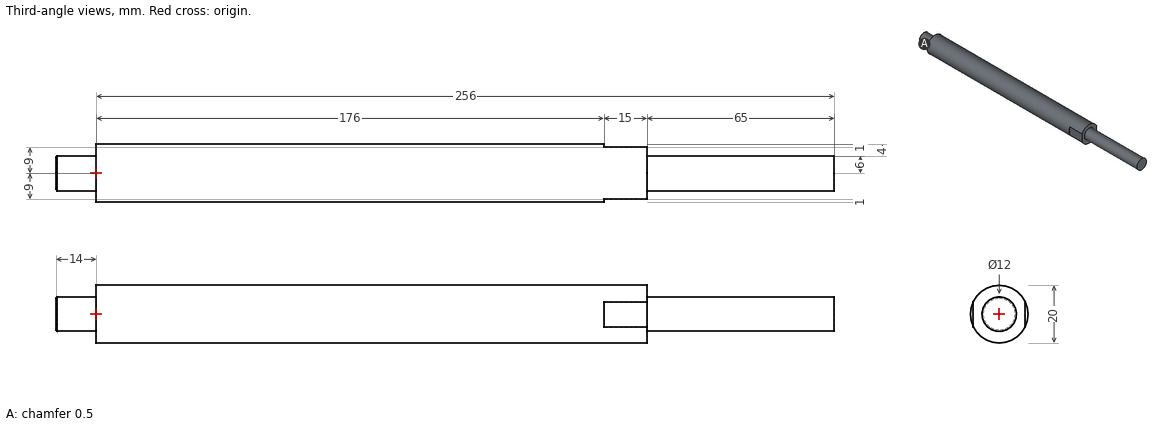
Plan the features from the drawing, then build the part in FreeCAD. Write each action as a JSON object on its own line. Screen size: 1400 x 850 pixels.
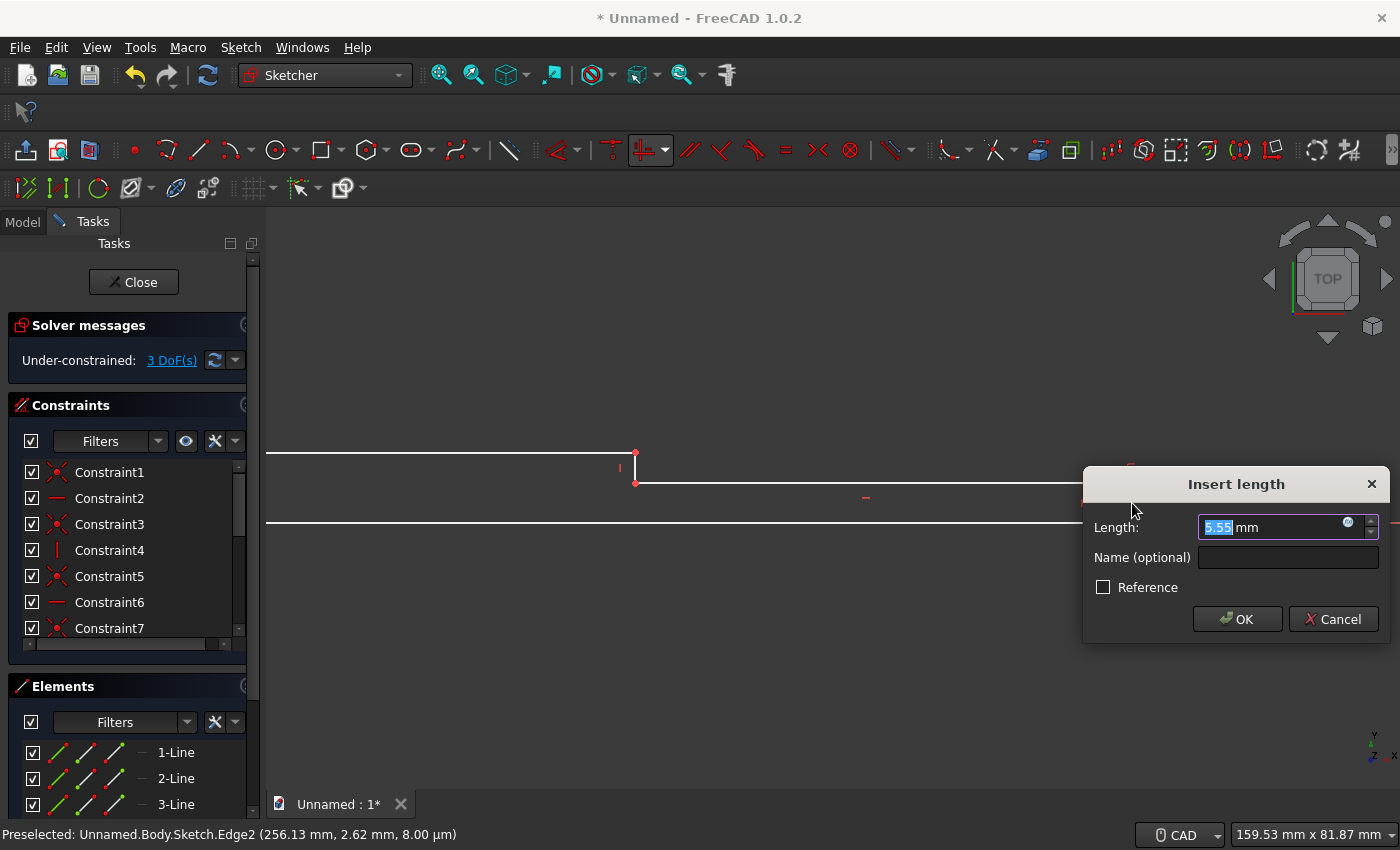
{"action": "type", "text": "6"}
{"action": "key", "text": "Return"}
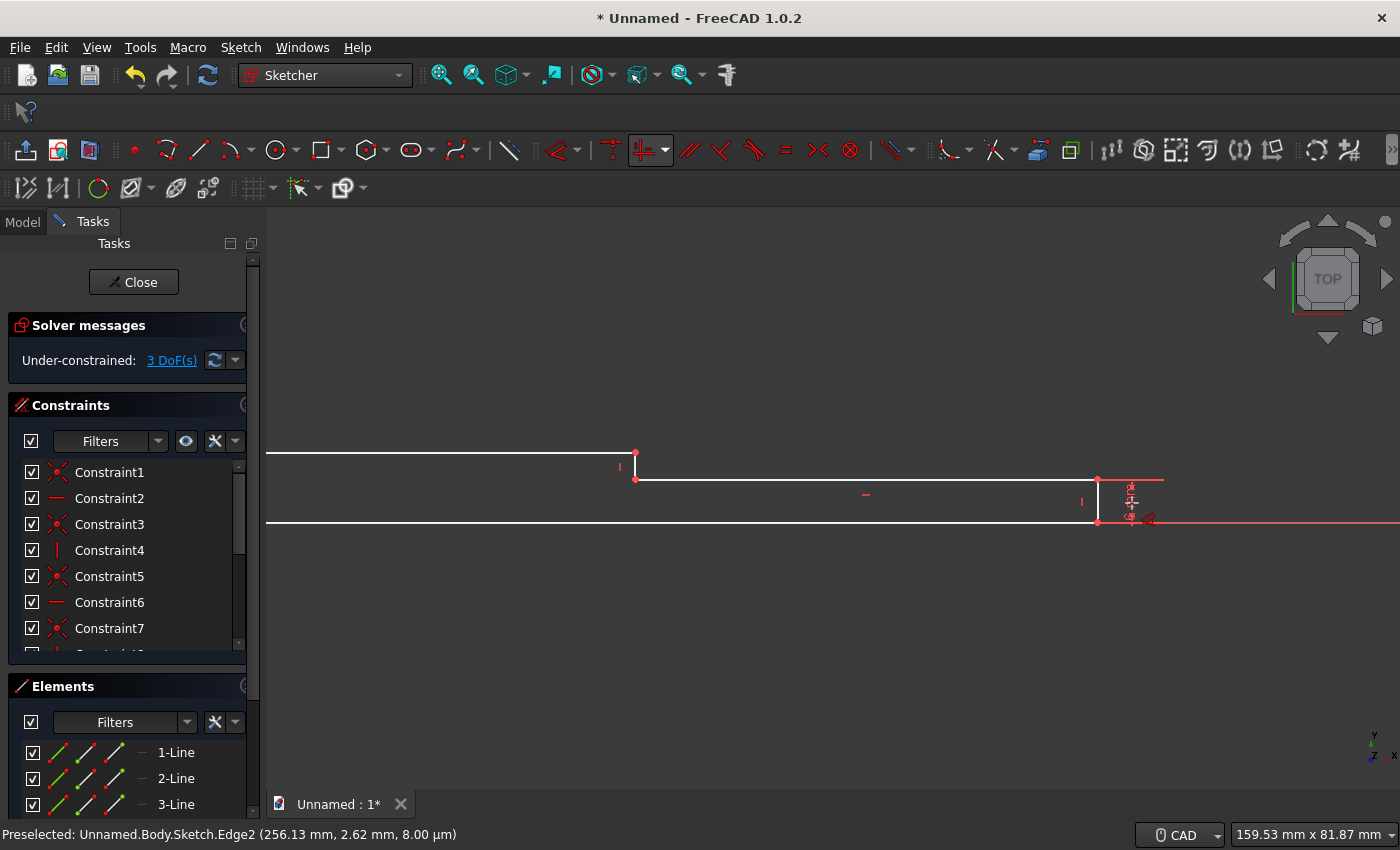
{"action": "scroll", "coordinate": [635, 469], "scroll_direction": "up", "scroll_amount": 2}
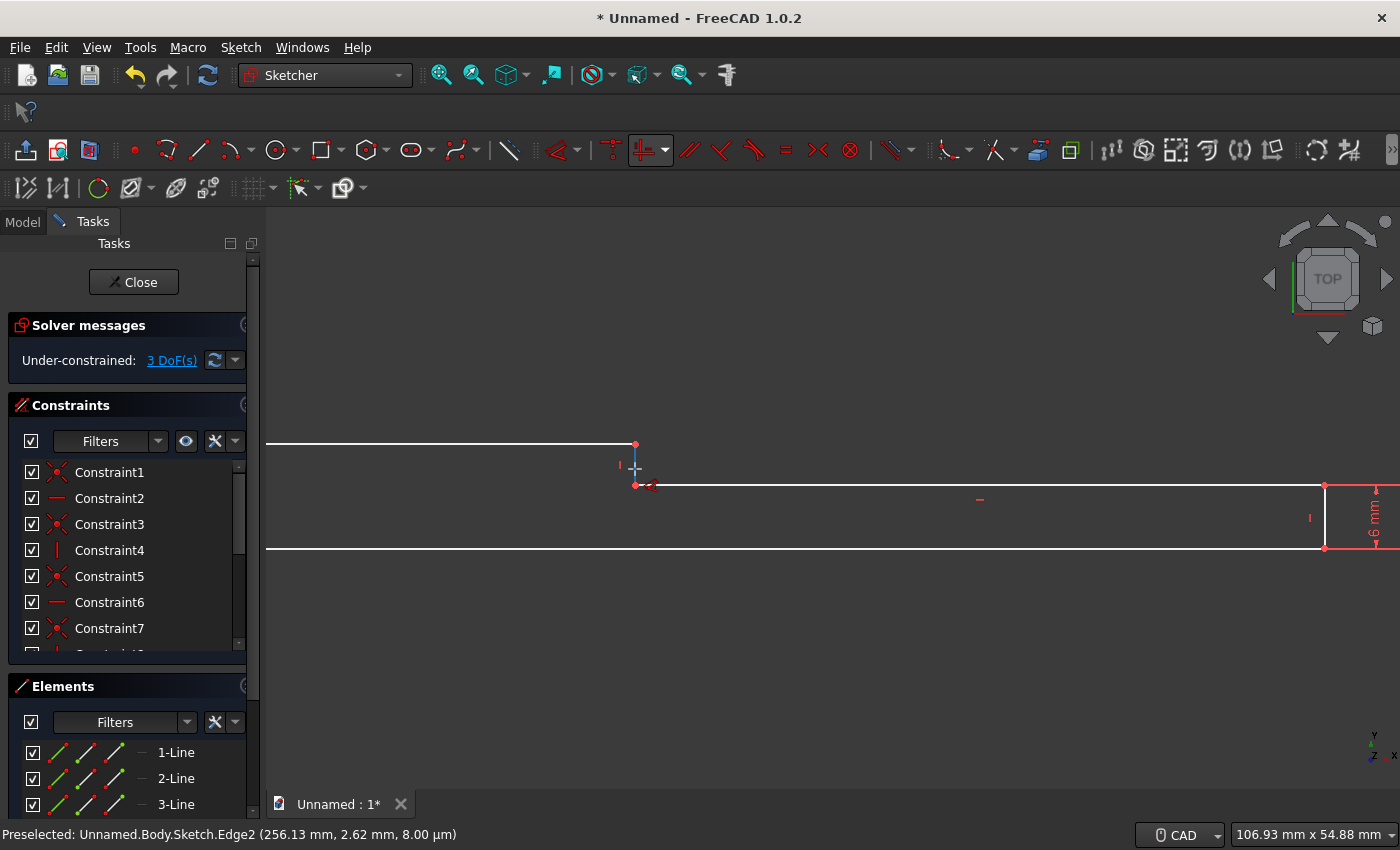
{"action": "left_click", "coordinate": [635, 469]}
{"action": "left_click", "coordinate": [669, 465]}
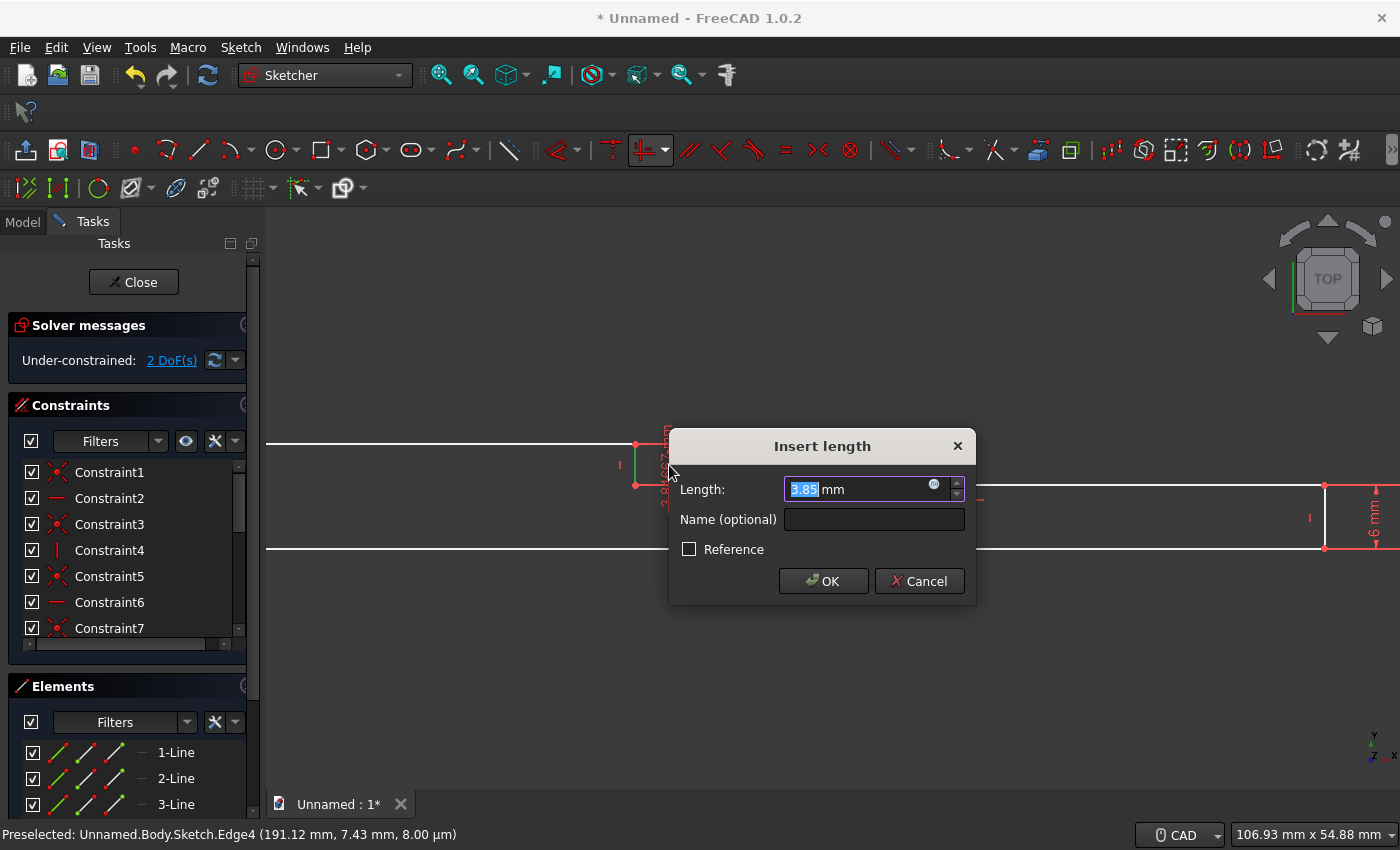
{"action": "type", "text": "4"}
{"action": "key", "text": "Return"}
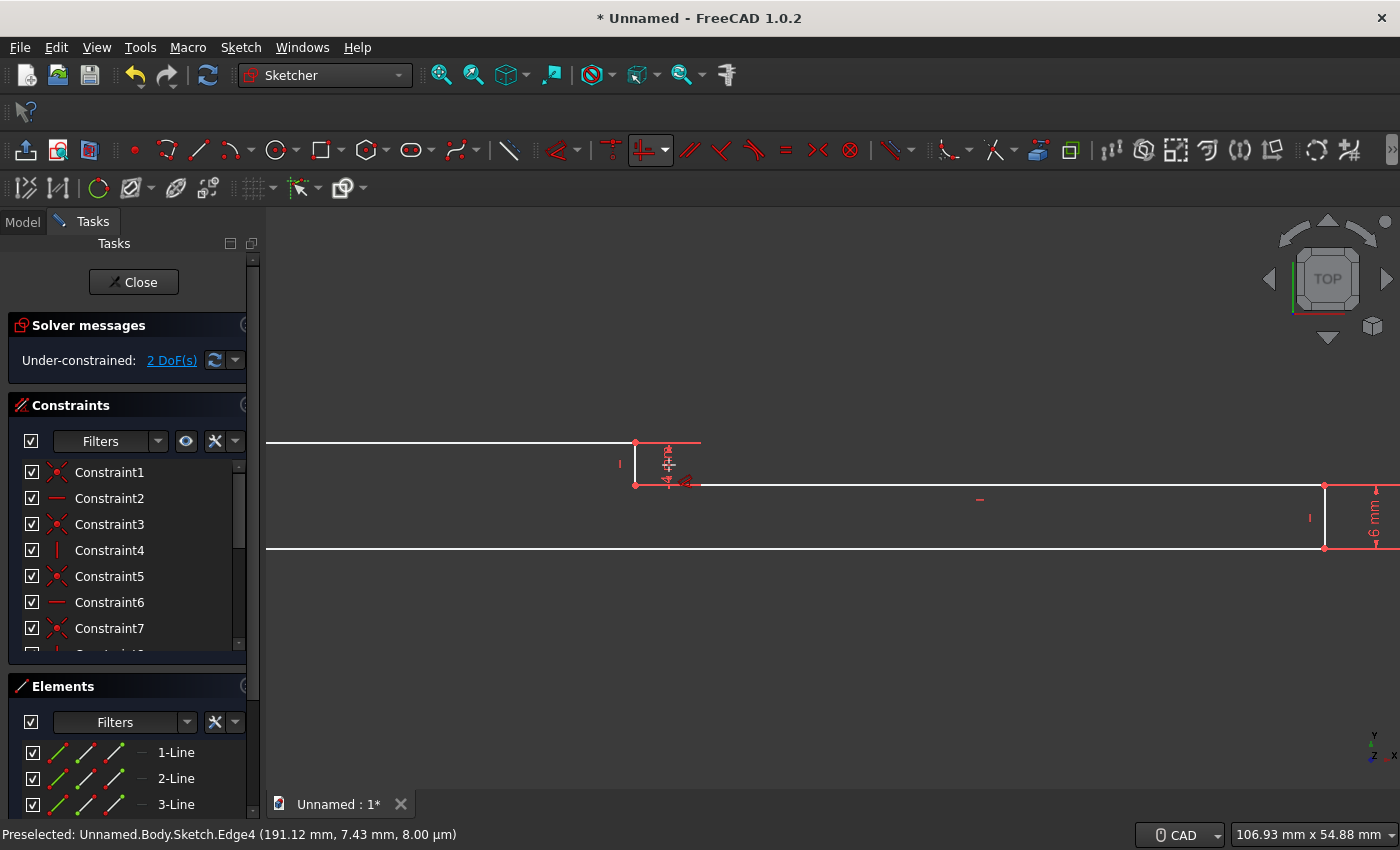
{"action": "scroll", "coordinate": [1026, 499], "scroll_direction": "down", "scroll_amount": 7}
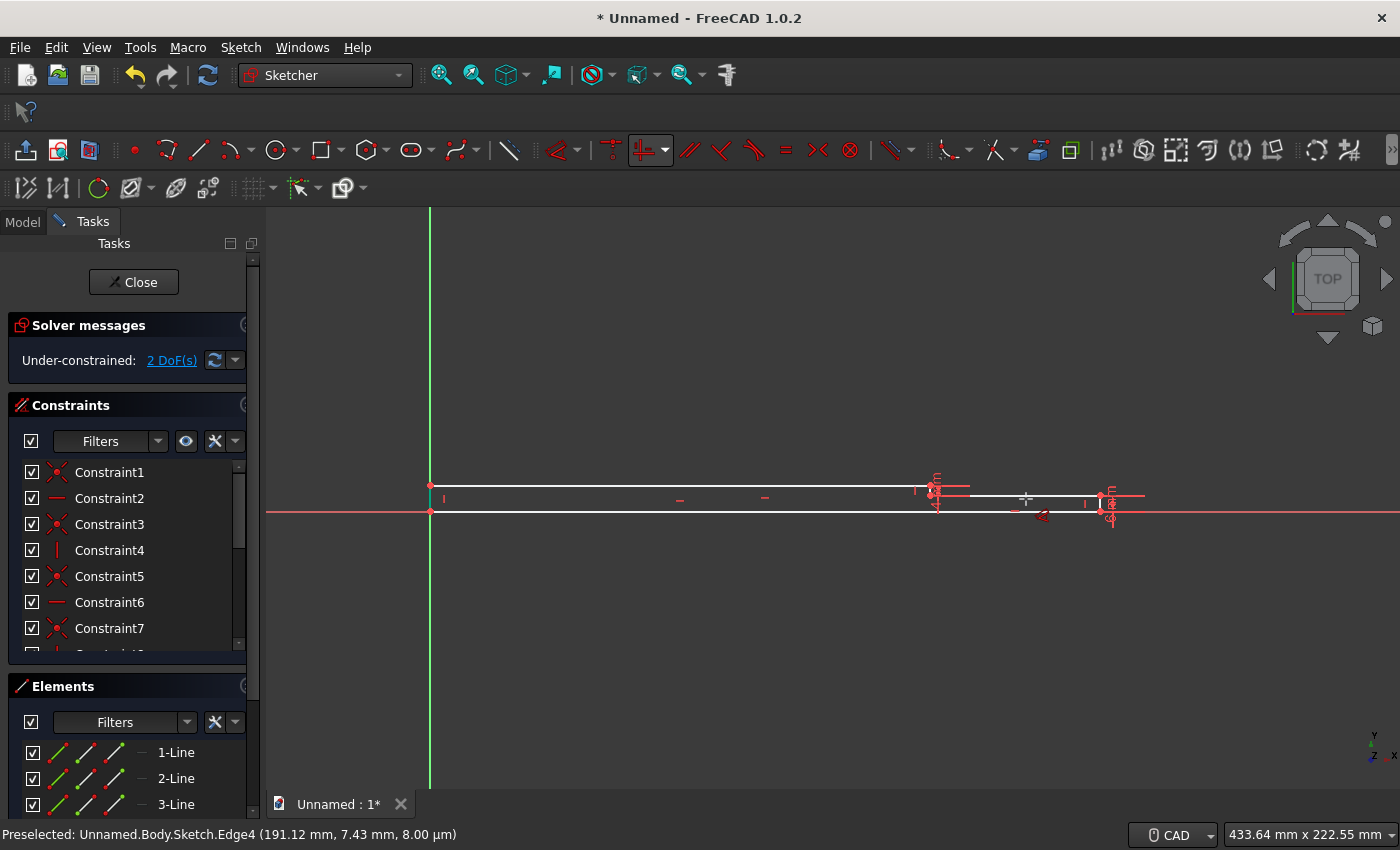
{"action": "left_click", "coordinate": [1049, 496]}
{"action": "left_click", "coordinate": [1015, 462]}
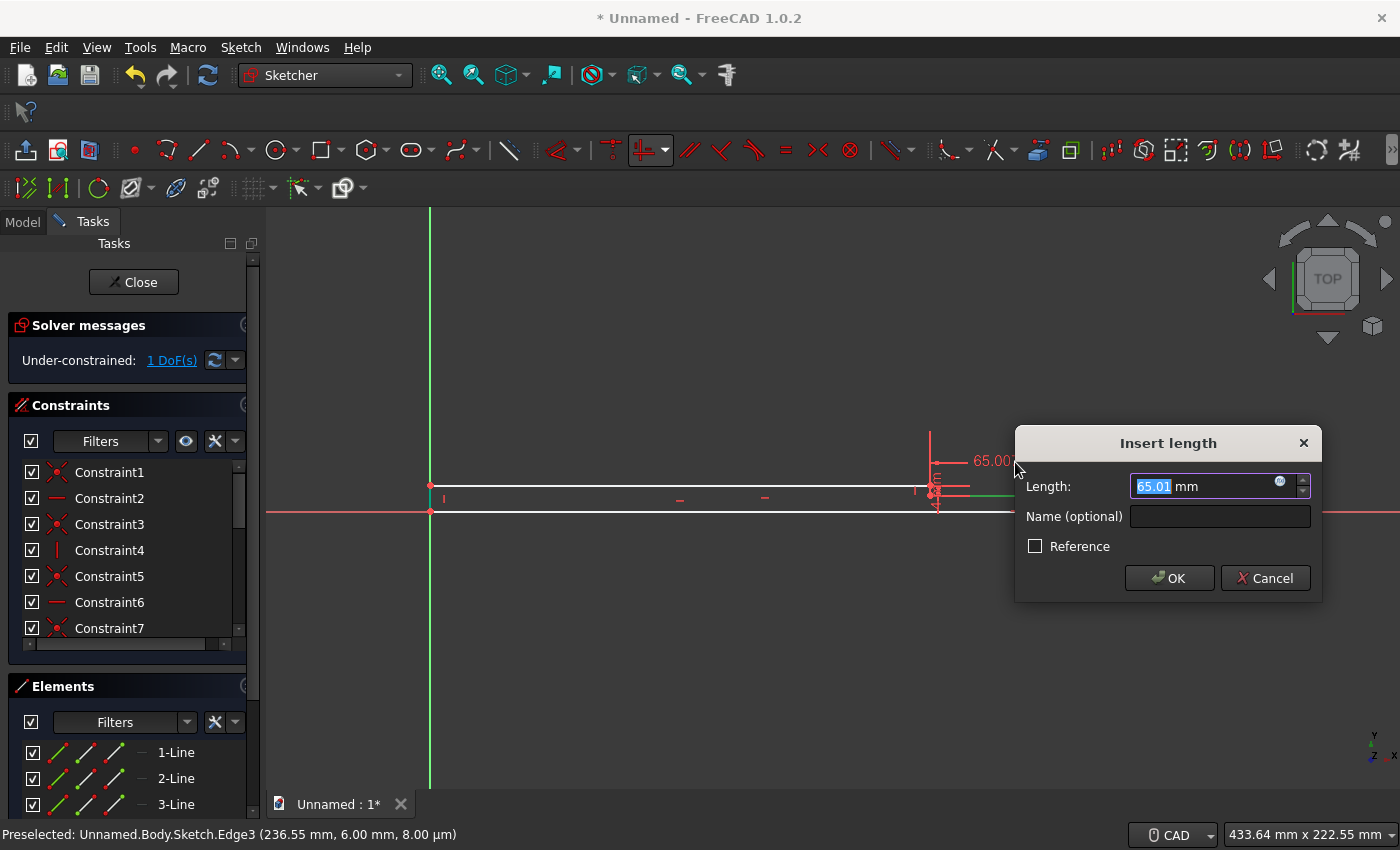
{"action": "type", "text": "65"}
{"action": "key", "text": "Return"}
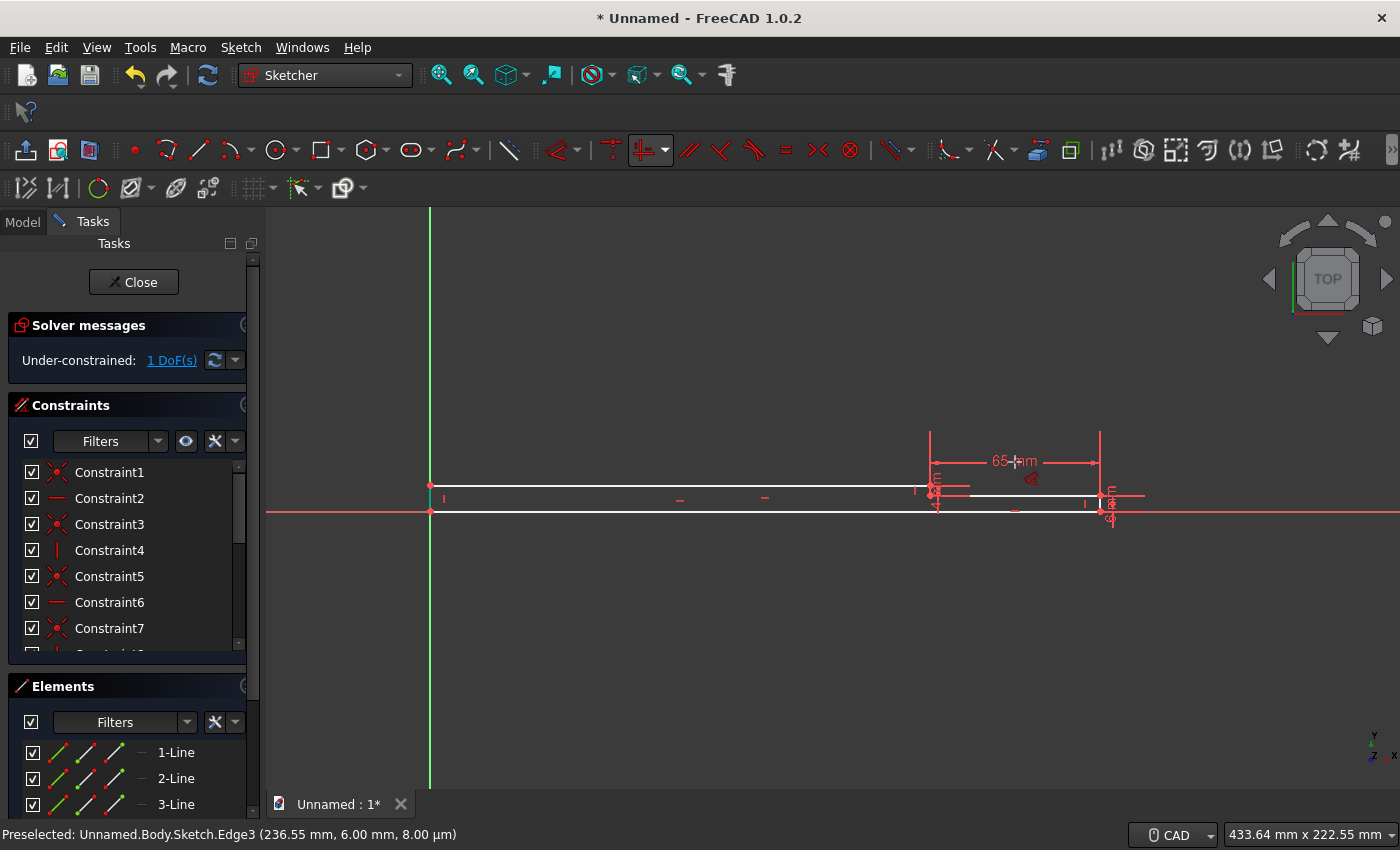
{"action": "left_click", "coordinate": [631, 512]}
{"action": "left_click", "coordinate": [765, 546]}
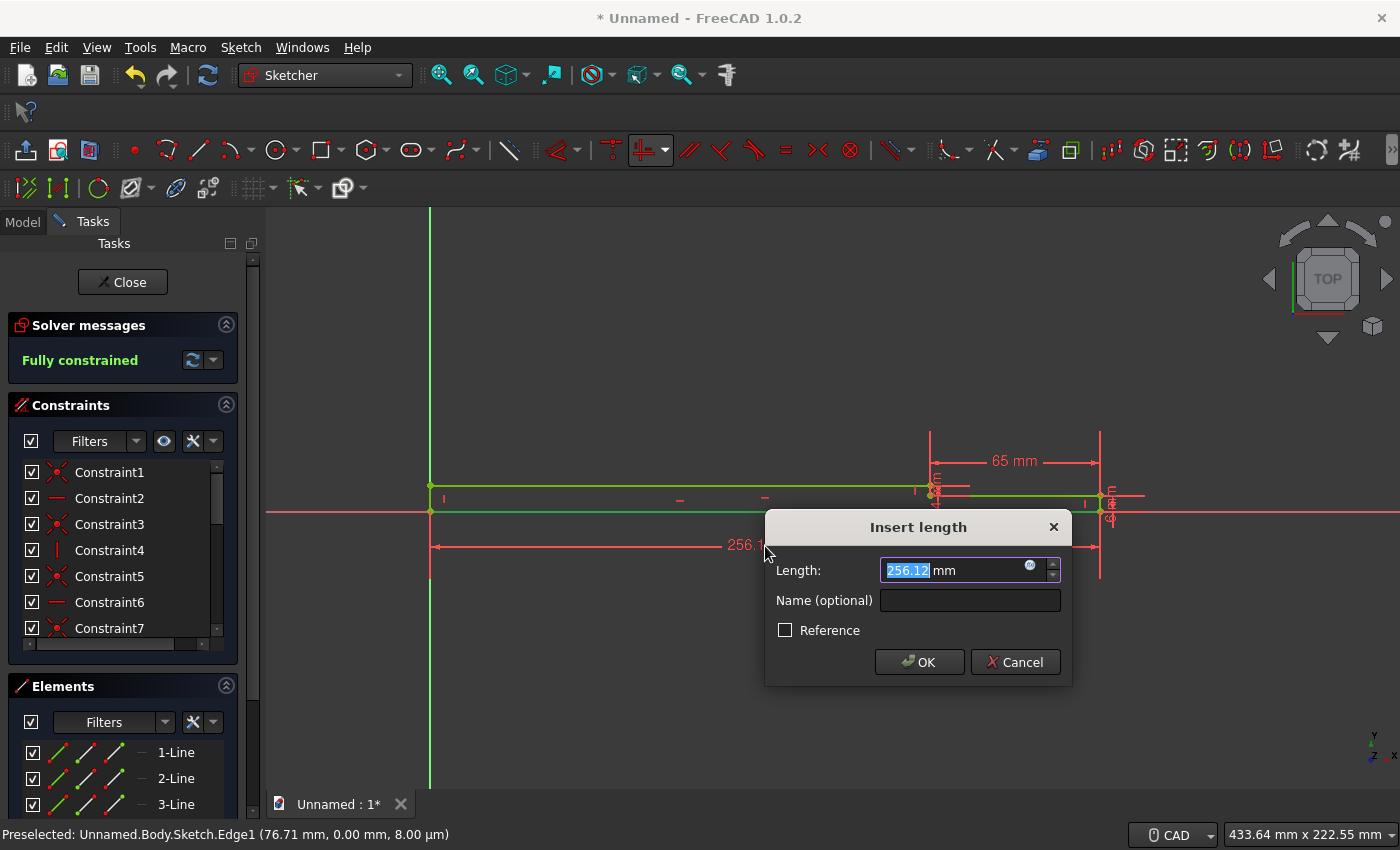
{"action": "type", "text": "256"}
{"action": "key", "text": "Return"}
{"action": "key", "text": "Escape"}